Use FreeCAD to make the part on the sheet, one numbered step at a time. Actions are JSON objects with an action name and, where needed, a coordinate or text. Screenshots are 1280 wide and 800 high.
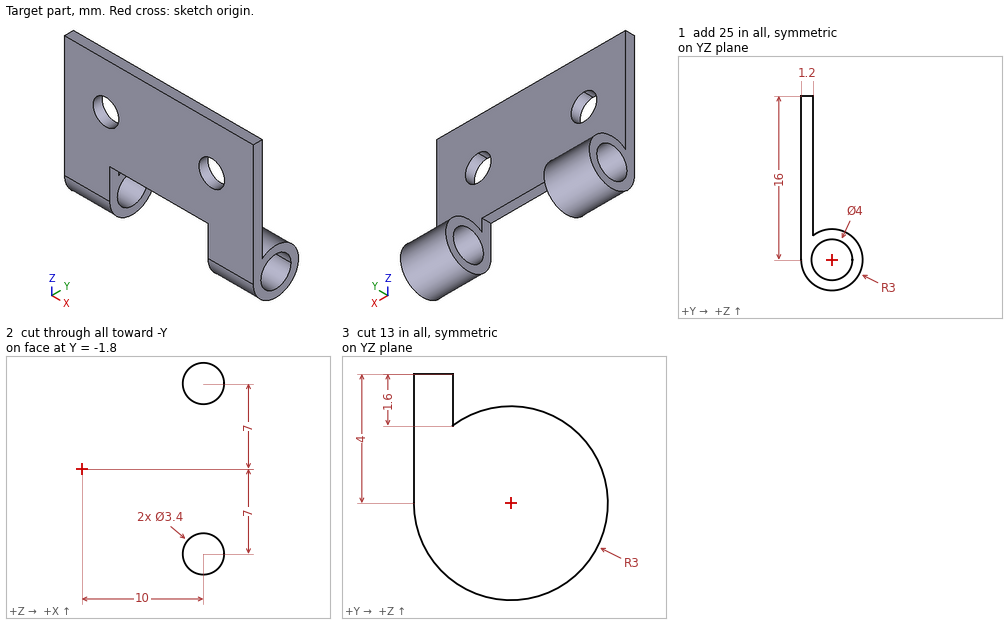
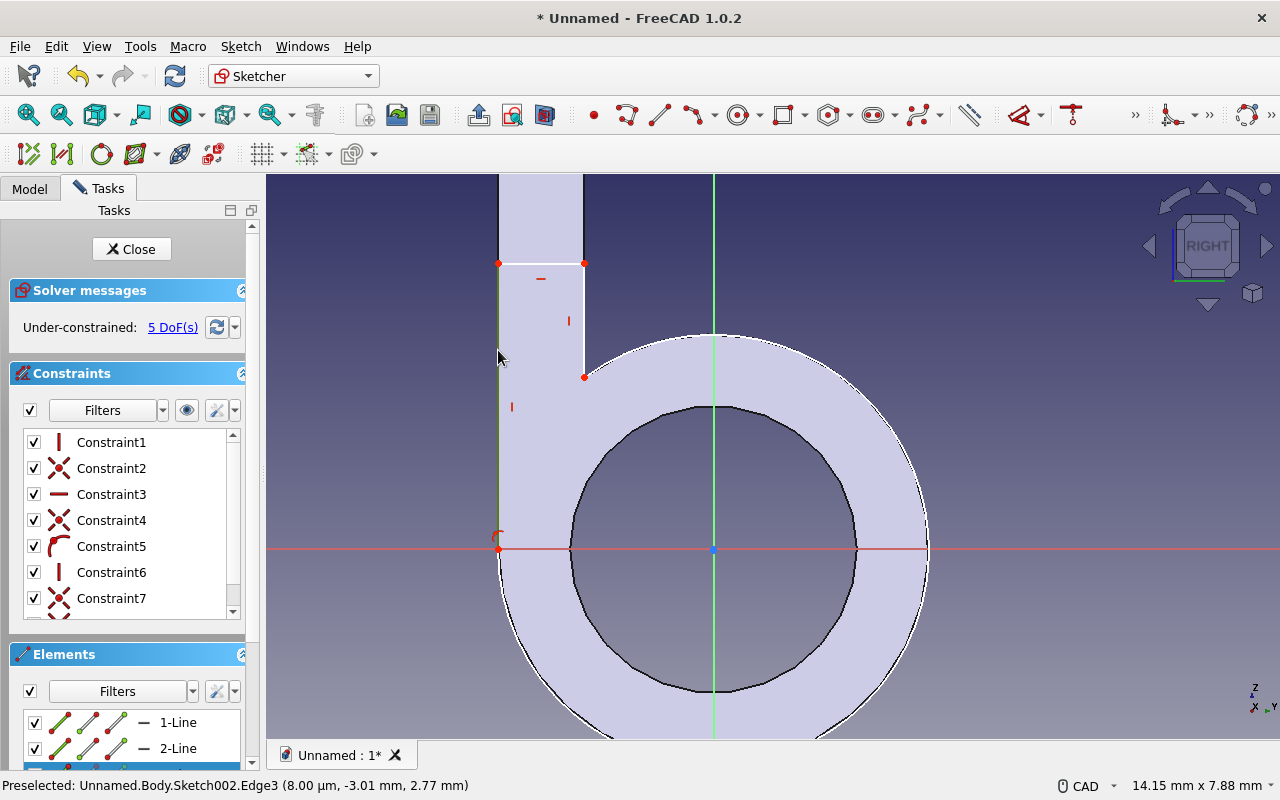
{"action": "left_click", "coordinate": [890, 427]}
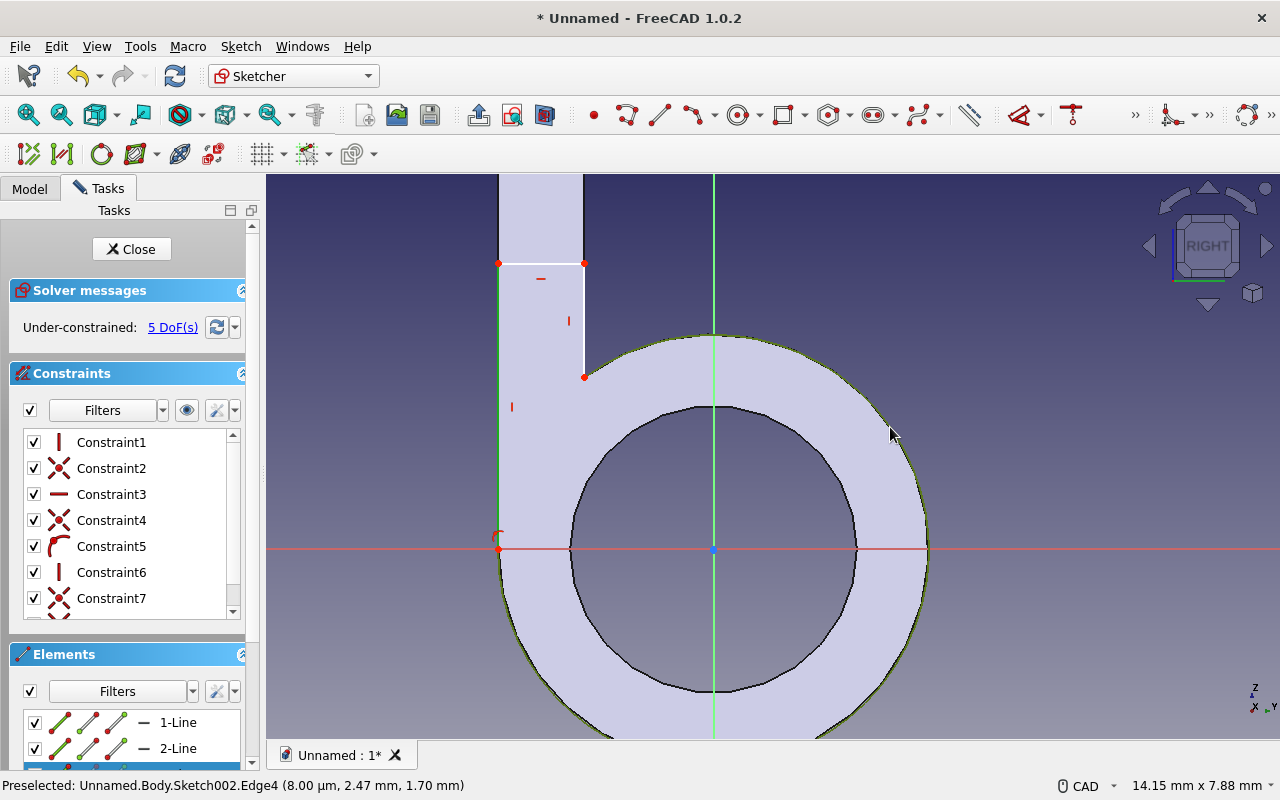
{"action": "key", "text": "t"}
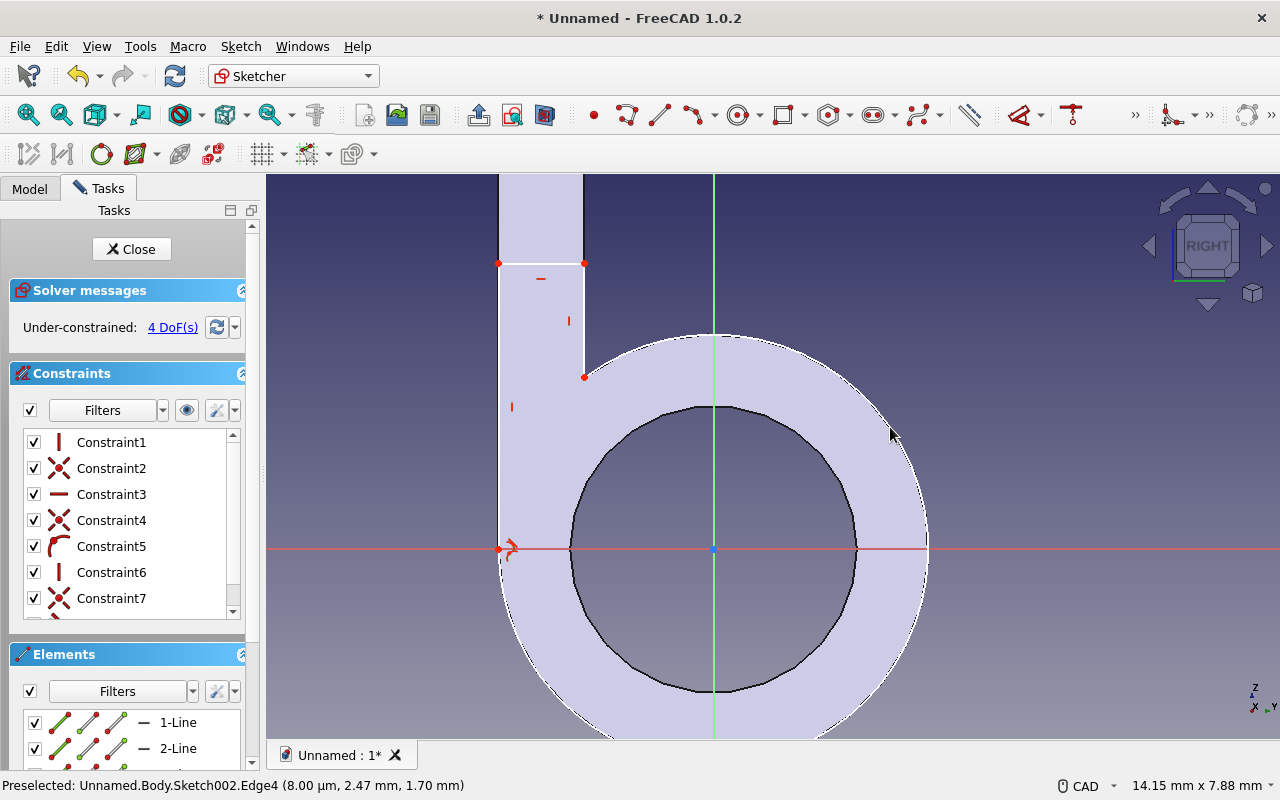
{"action": "left_click", "coordinate": [713, 549]}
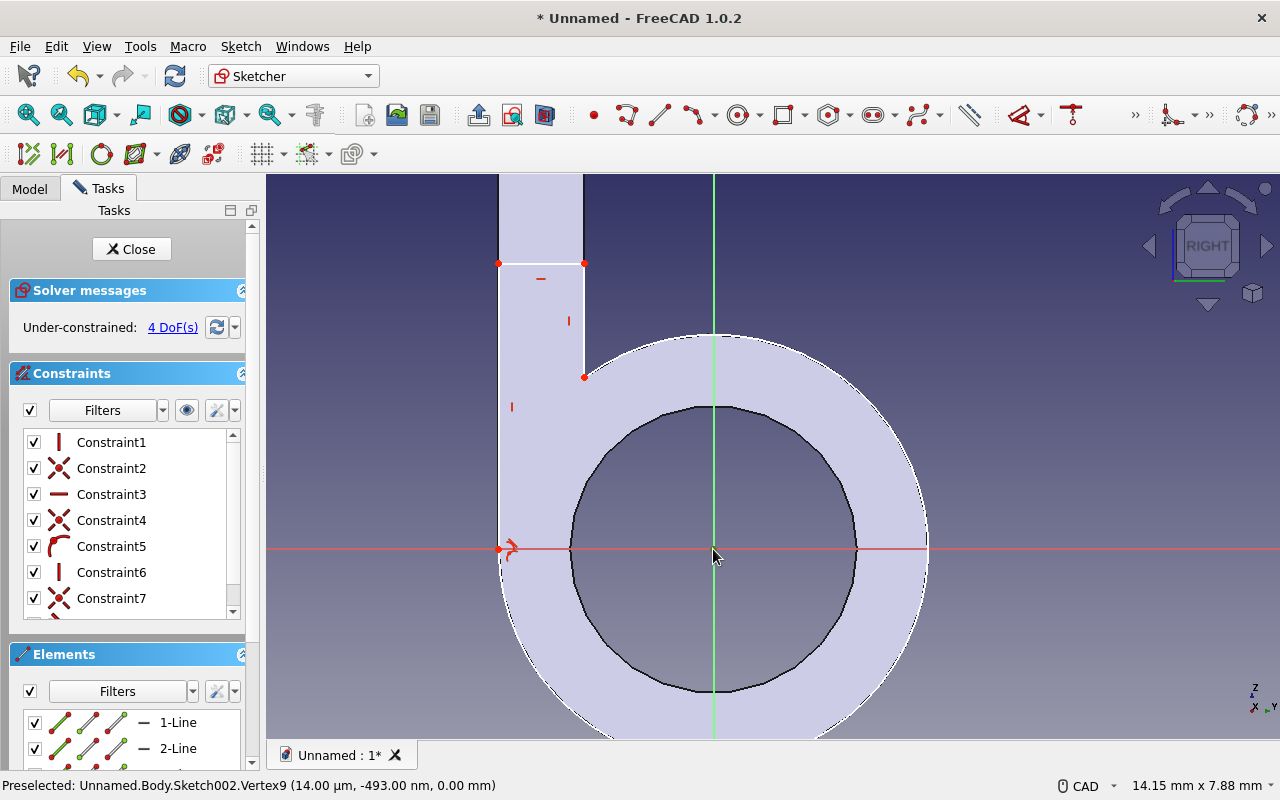
{"action": "left_click", "coordinate": [714, 675]}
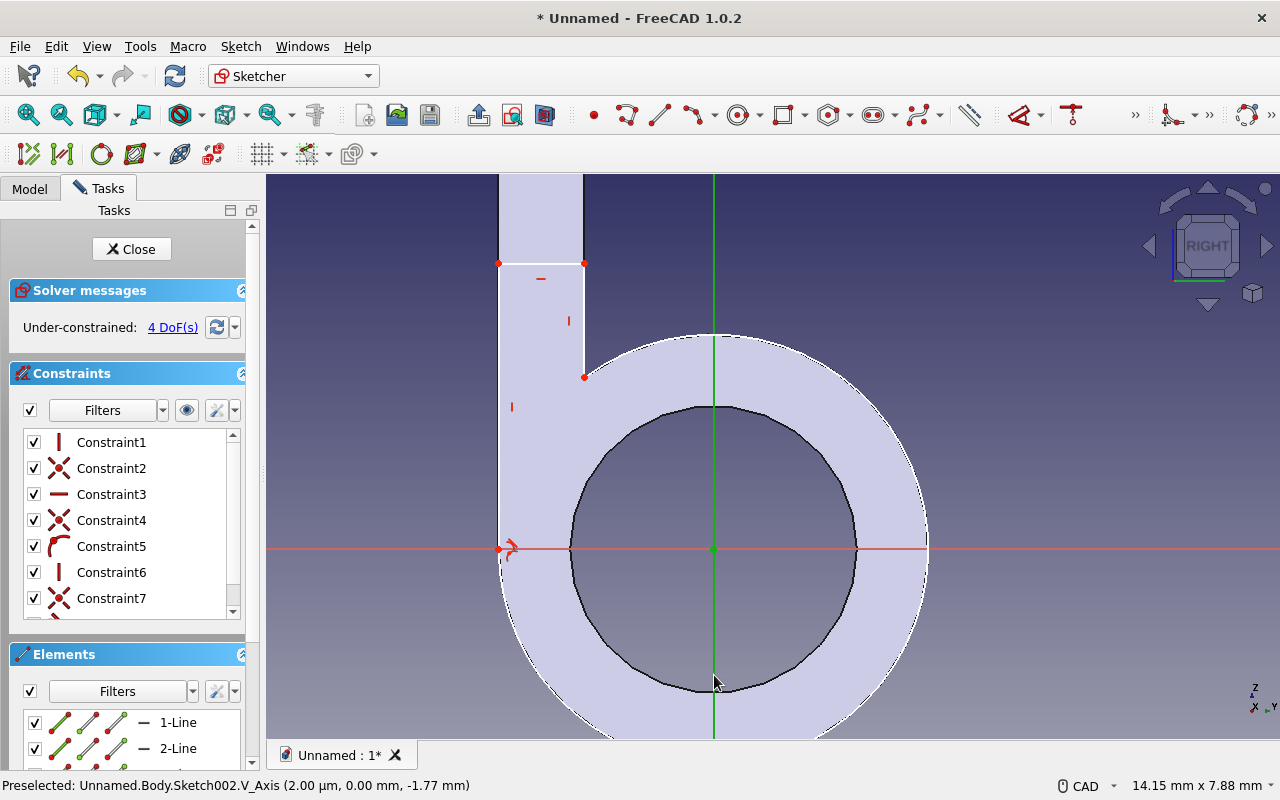
{"action": "left_click", "coordinate": [1071, 116]}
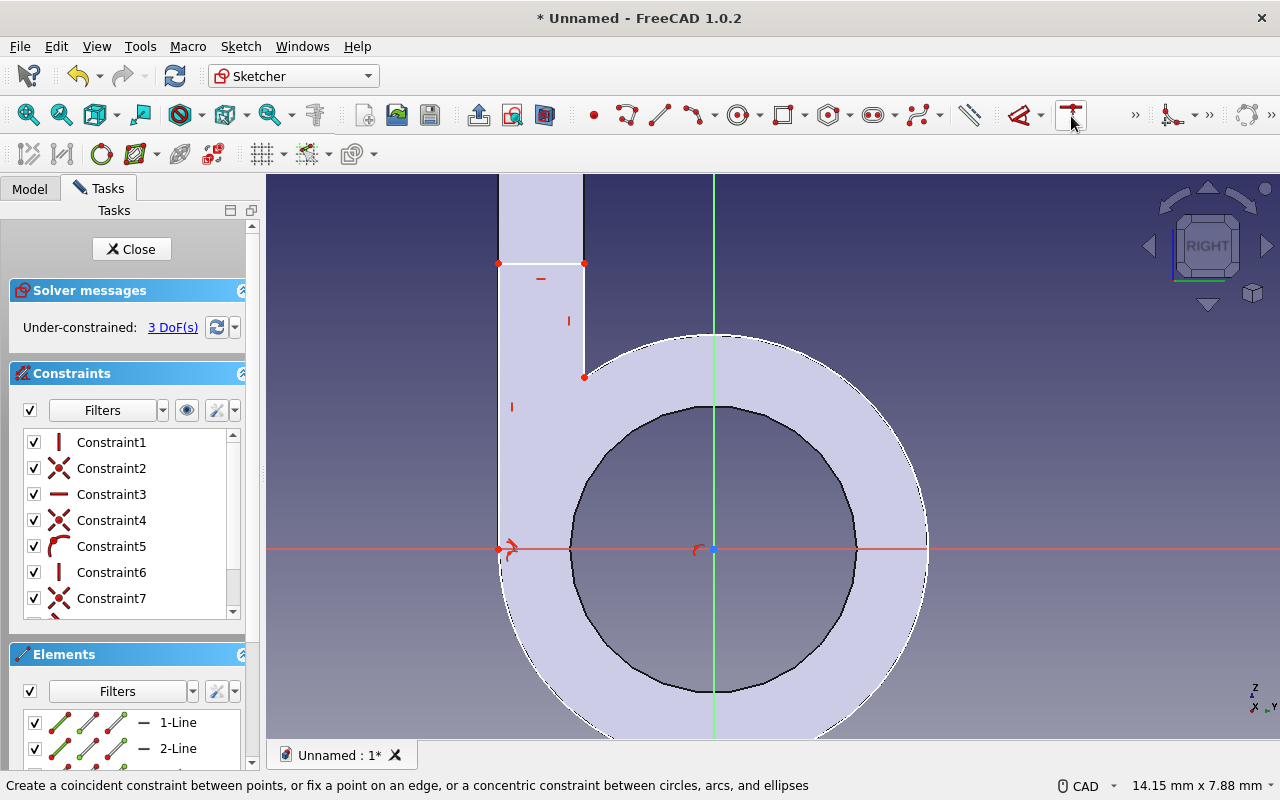
{"action": "left_click", "coordinate": [1018, 116]}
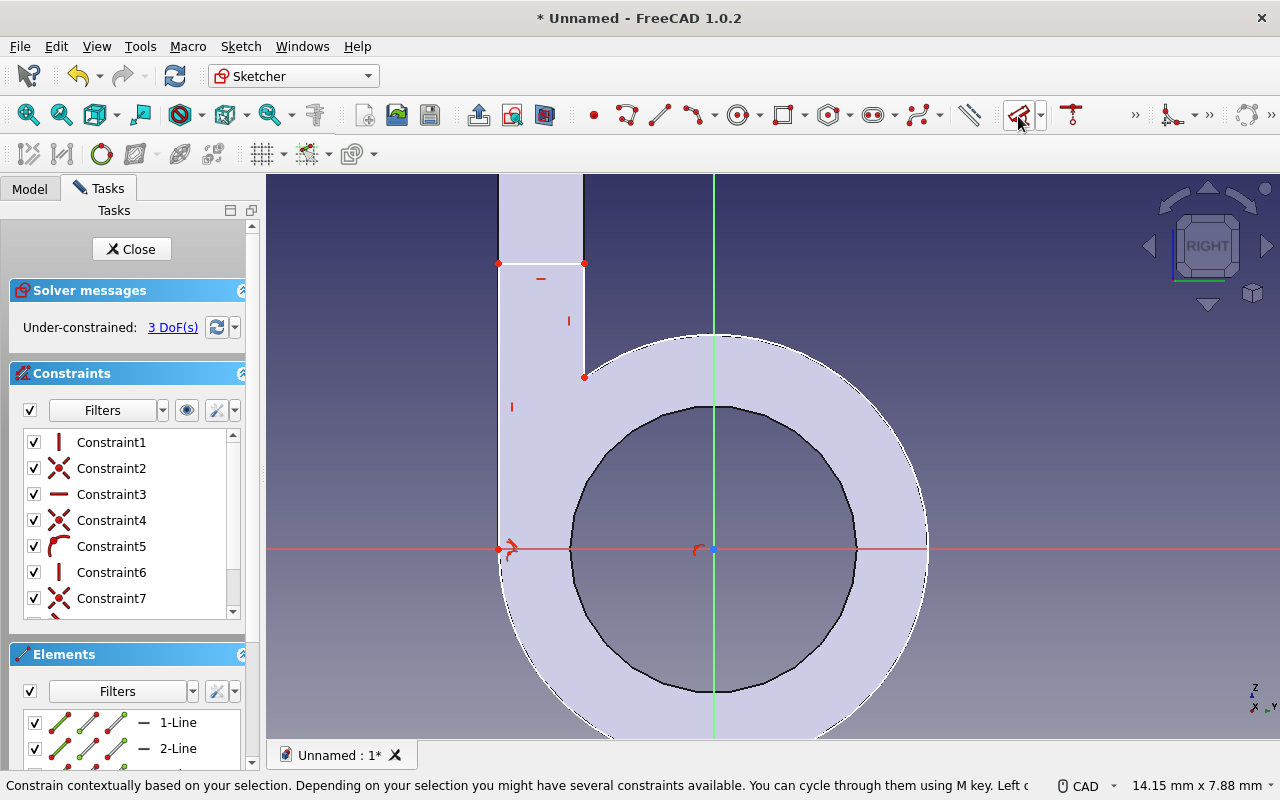
{"action": "left_click", "coordinate": [890, 426]}
{"action": "left_click", "coordinate": [916, 408]}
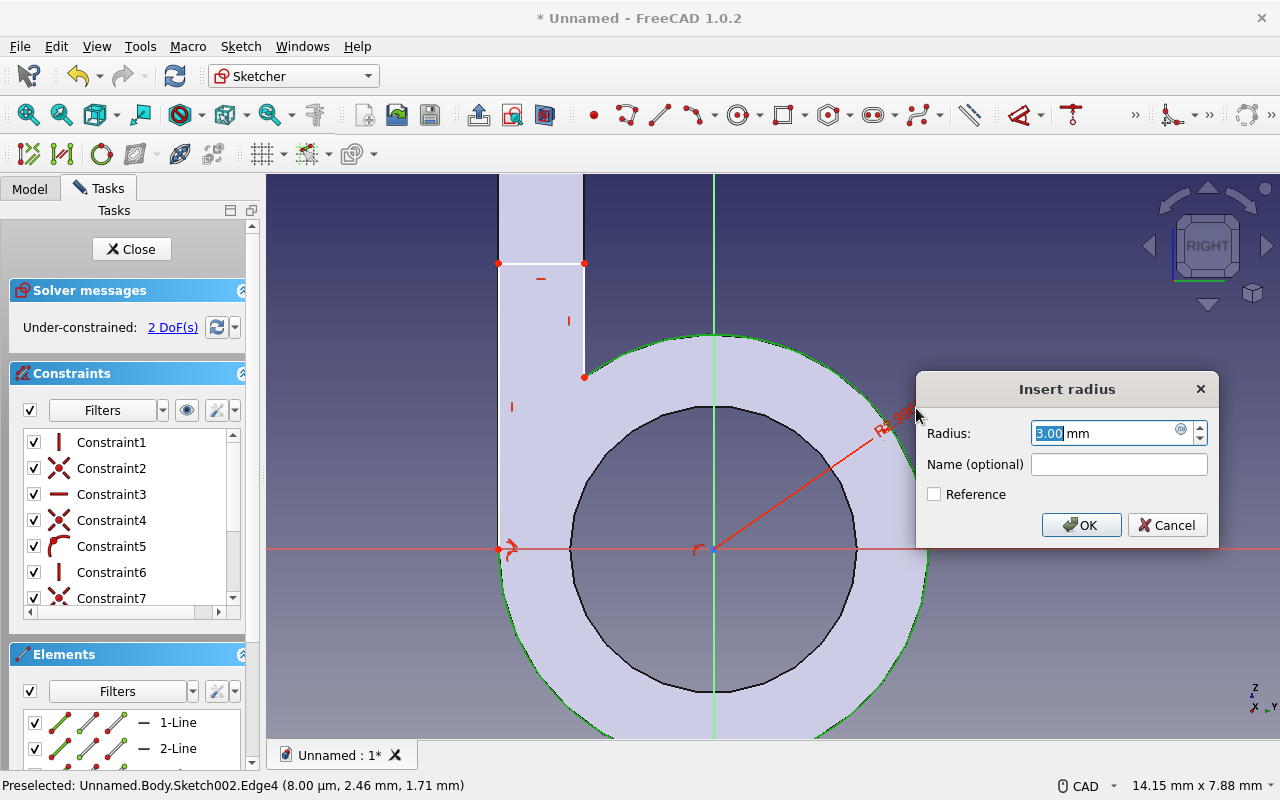
{"action": "type", "text": "3"}
{"action": "key", "text": "Return"}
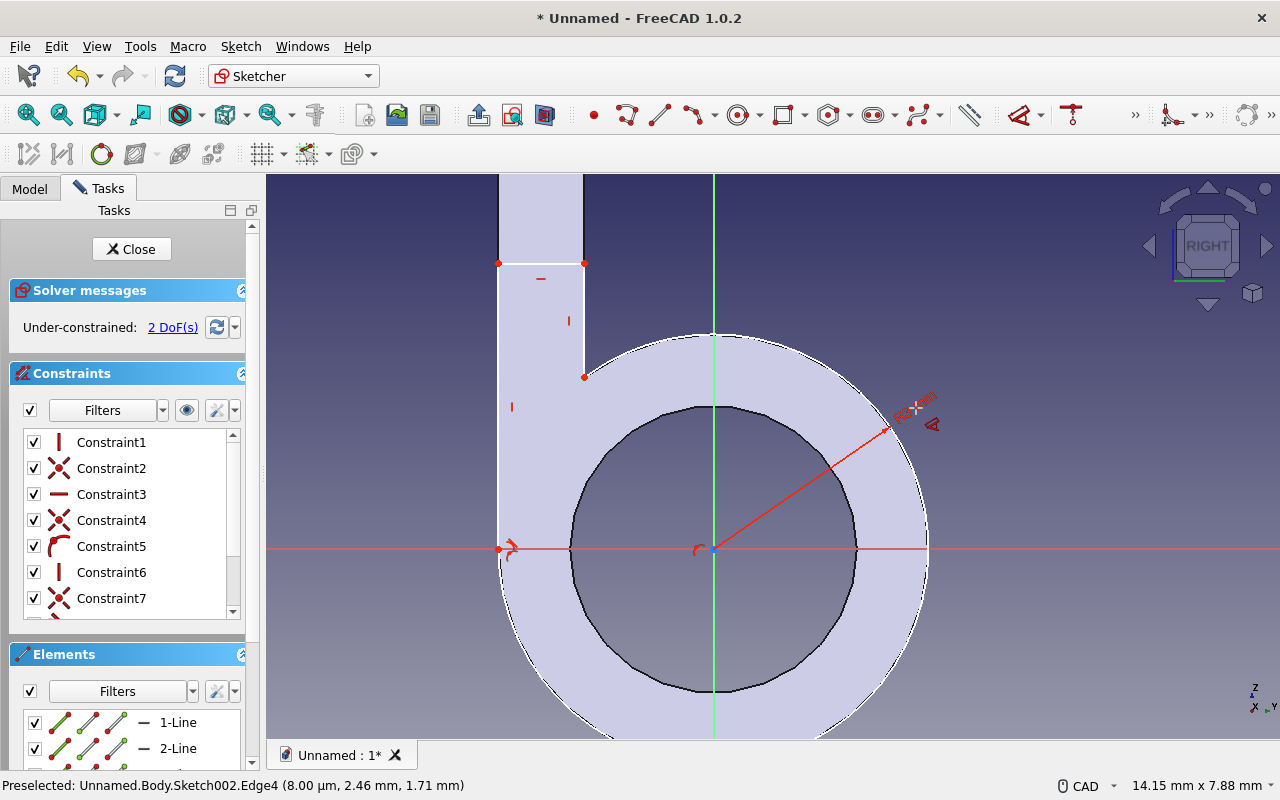
{"action": "left_click", "coordinate": [498, 350]}
{"action": "left_click", "coordinate": [464, 407]}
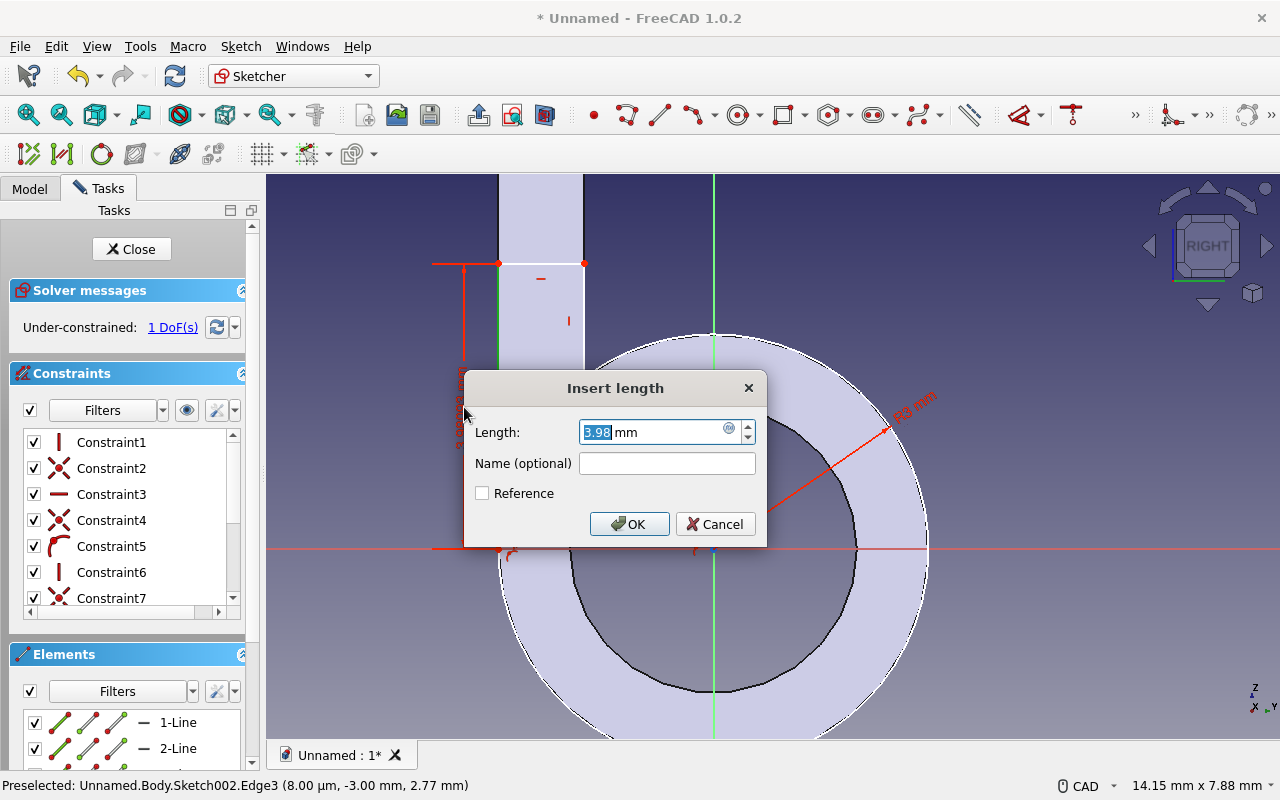
{"action": "type", "text": "4"}
{"action": "key", "text": "Return"}